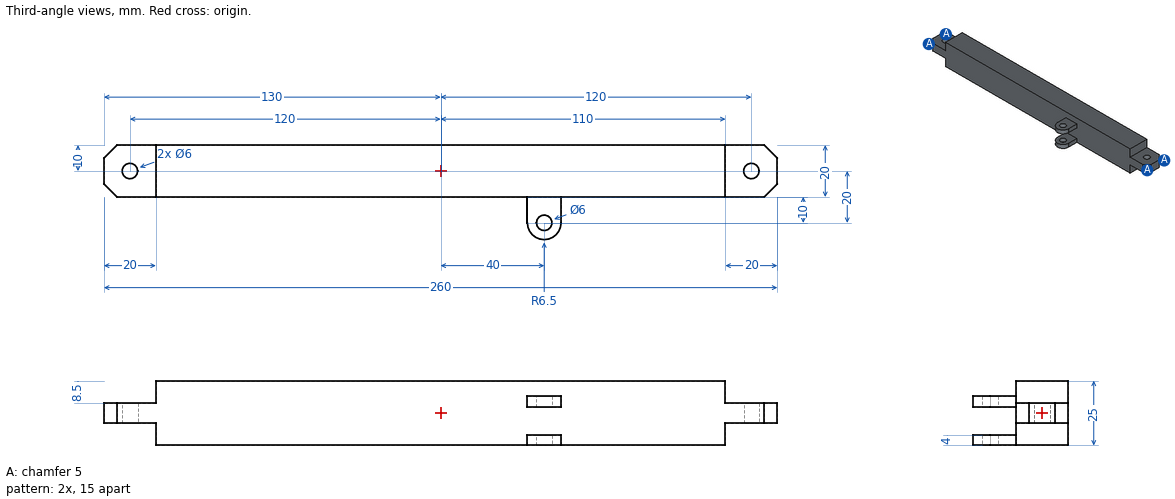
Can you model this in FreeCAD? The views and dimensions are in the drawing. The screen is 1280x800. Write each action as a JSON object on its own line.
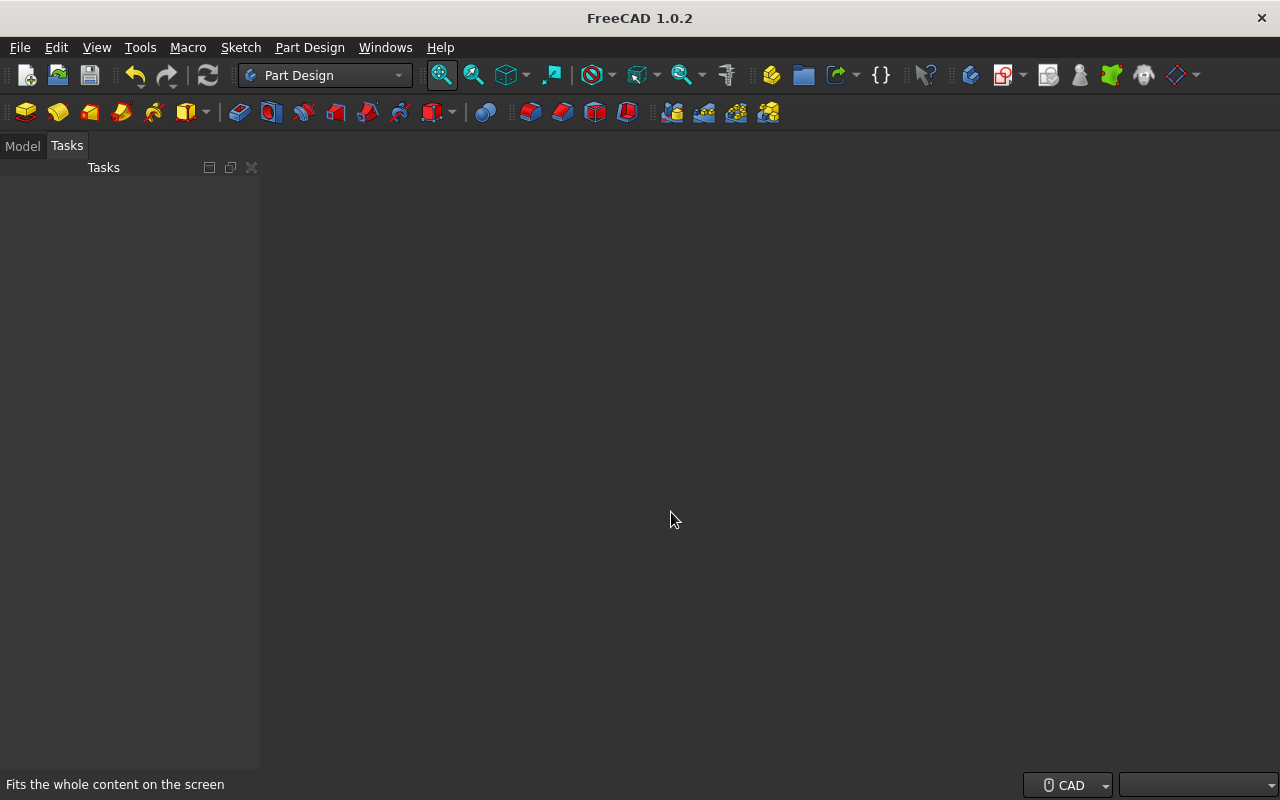
{"action": "key", "text": "ctrl+n"}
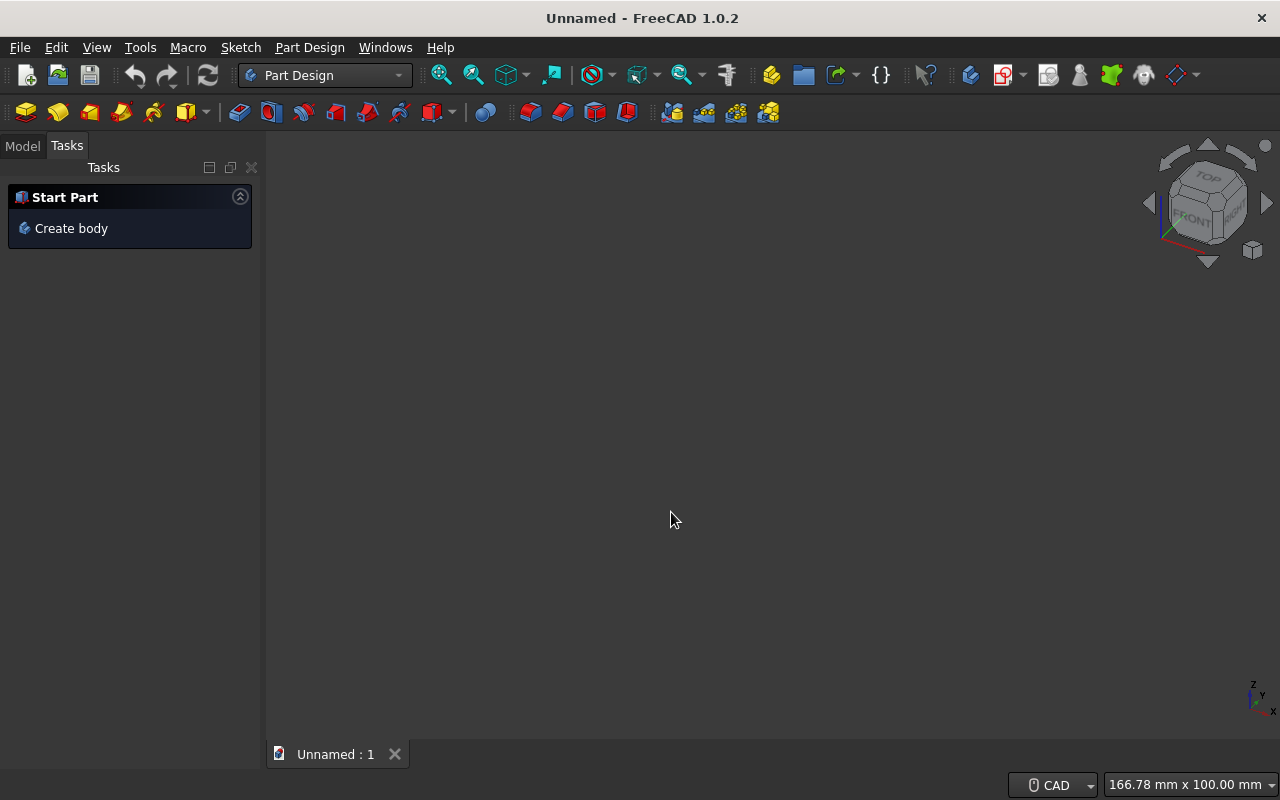
{"action": "left_click", "coordinate": [1004, 76]}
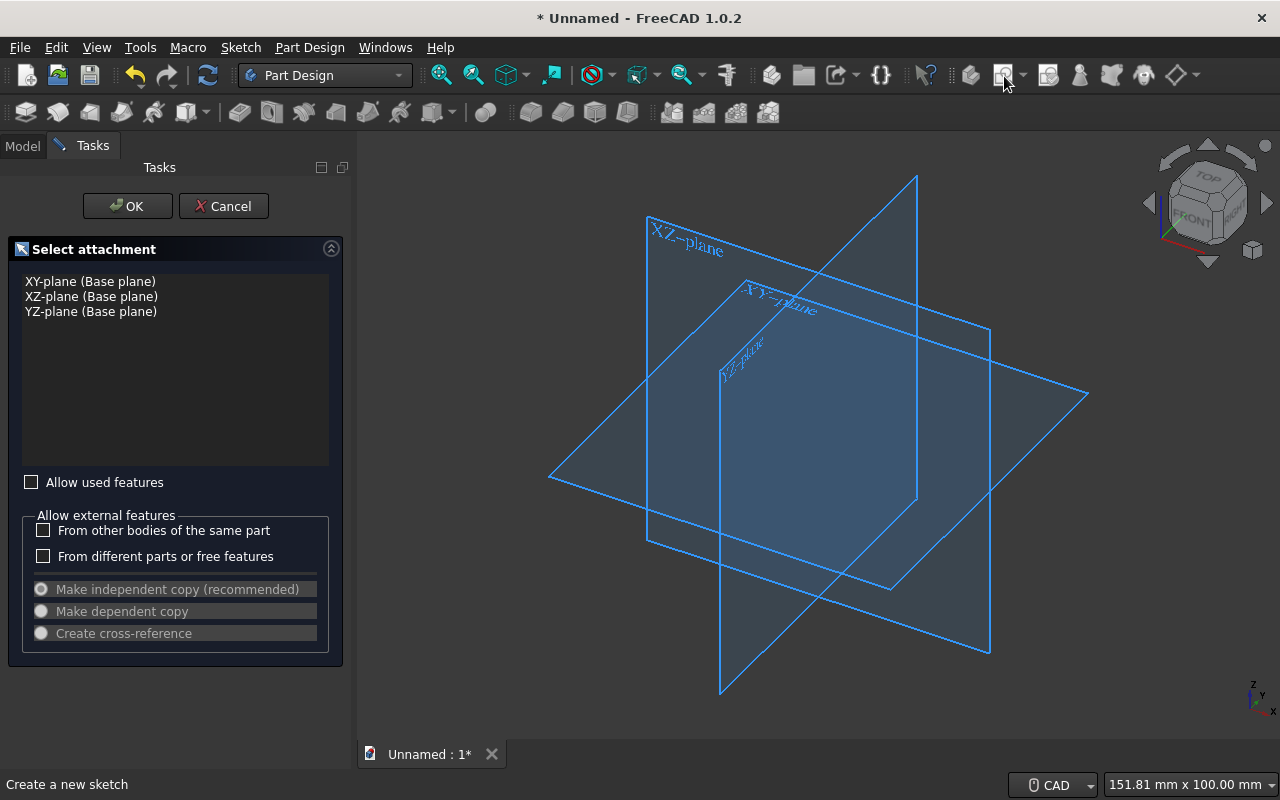
{"action": "left_click", "coordinate": [82, 282]}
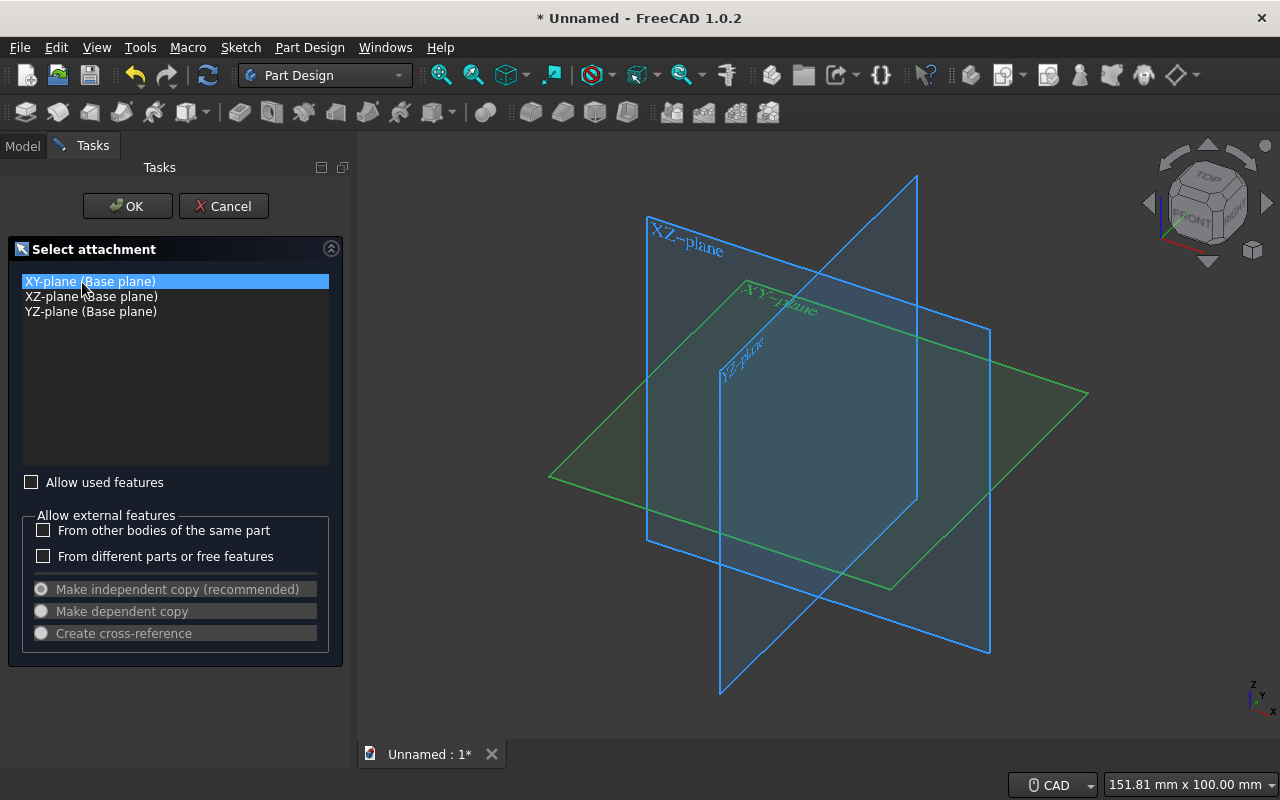
{"action": "left_click", "coordinate": [128, 206]}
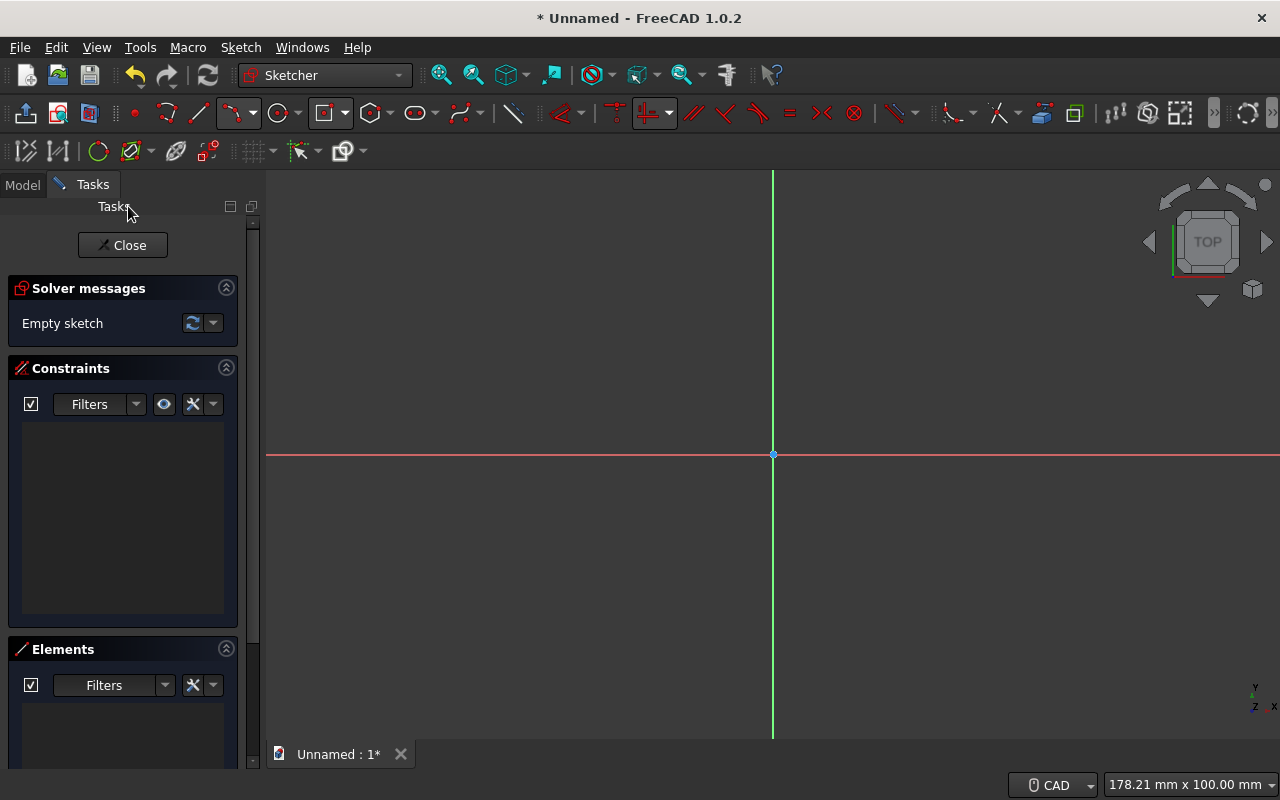
{"action": "scroll", "coordinate": [665, 454], "scroll_direction": "down", "scroll_amount": 5}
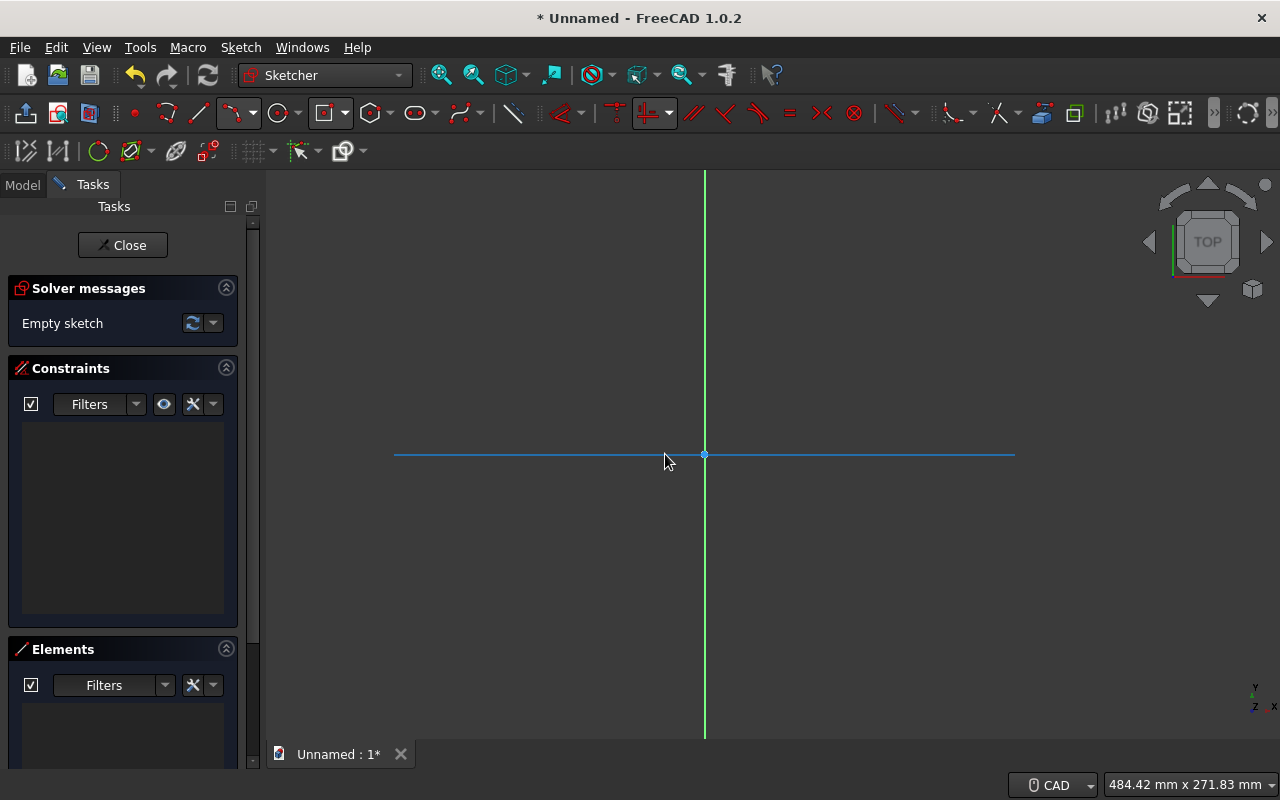
{"action": "key", "text": "g v"}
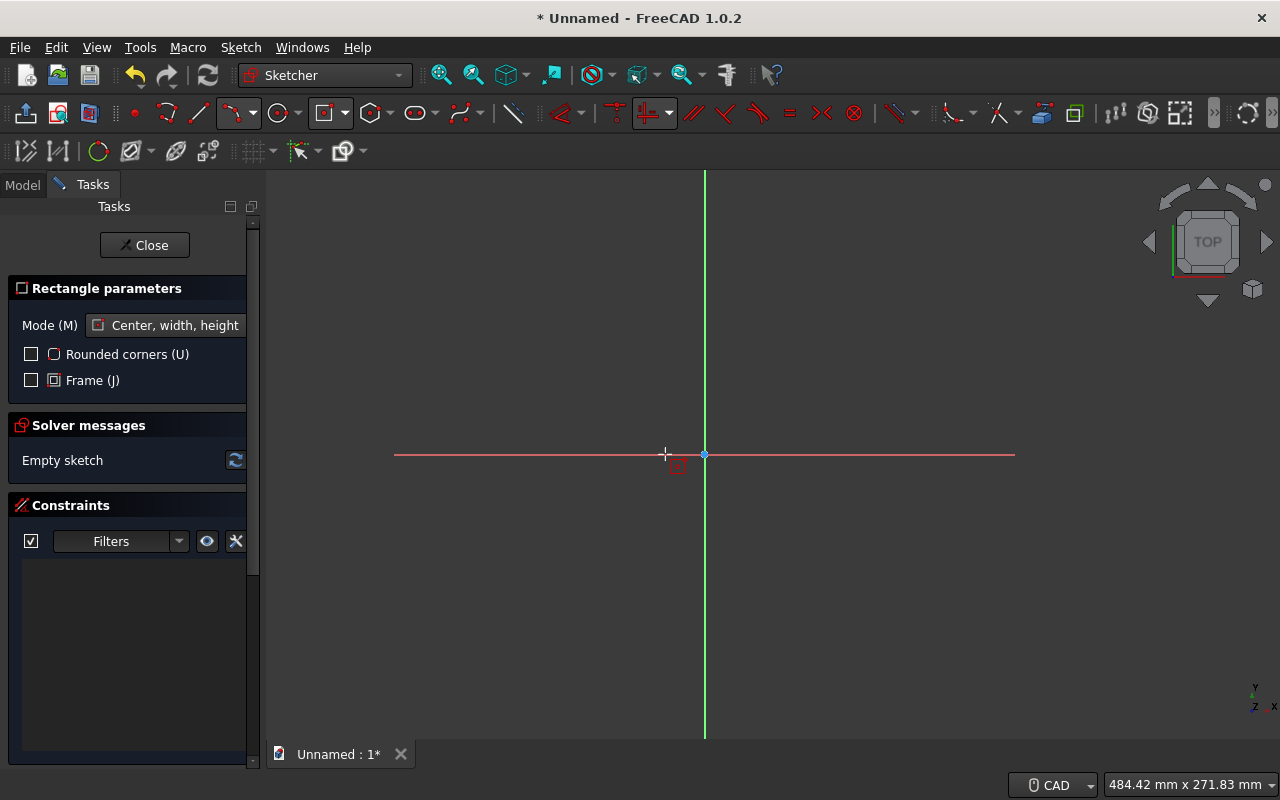
{"action": "left_click", "coordinate": [705, 454]}
{"action": "mouse_move", "coordinate": [977, 434]}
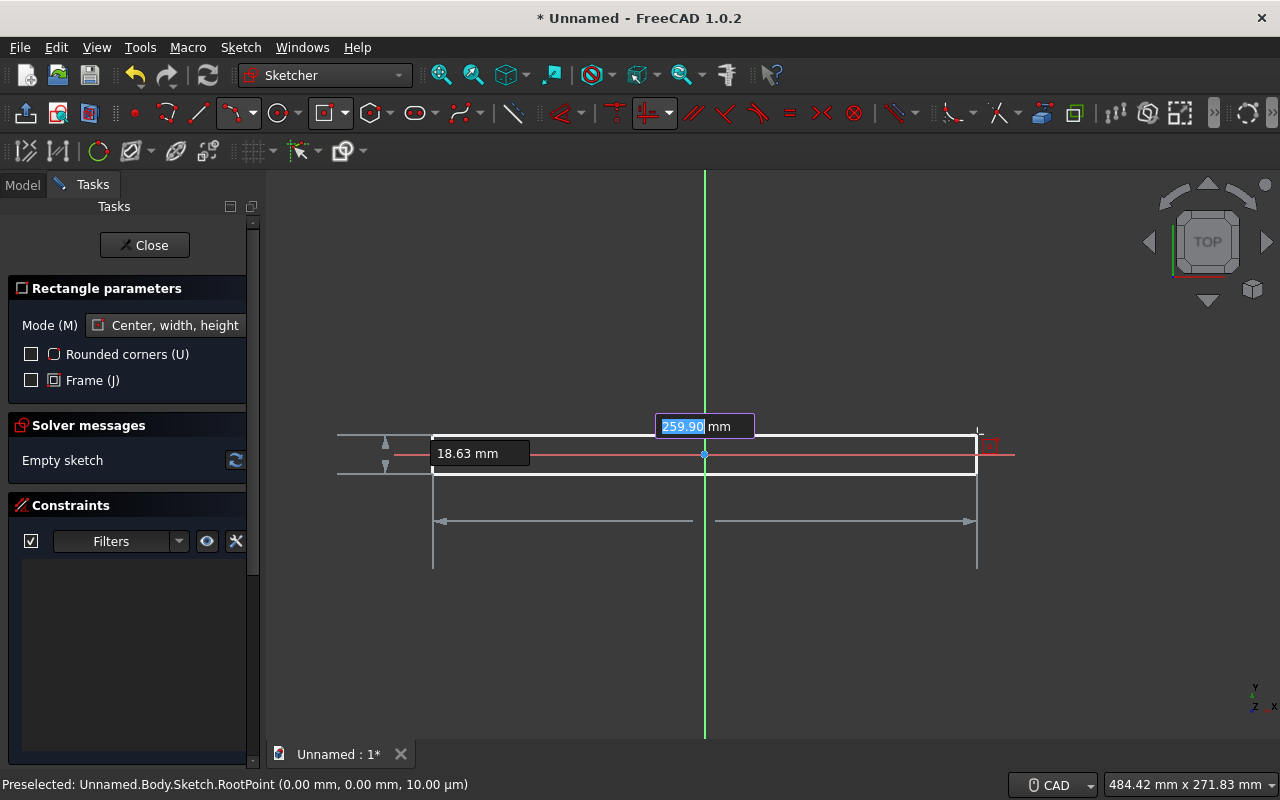
{"action": "type", "text": "260"}
{"action": "key", "text": "Tab"}
{"action": "type", "text": "20"}
{"action": "key", "text": "Return"}
{"action": "key", "text": "Escape"}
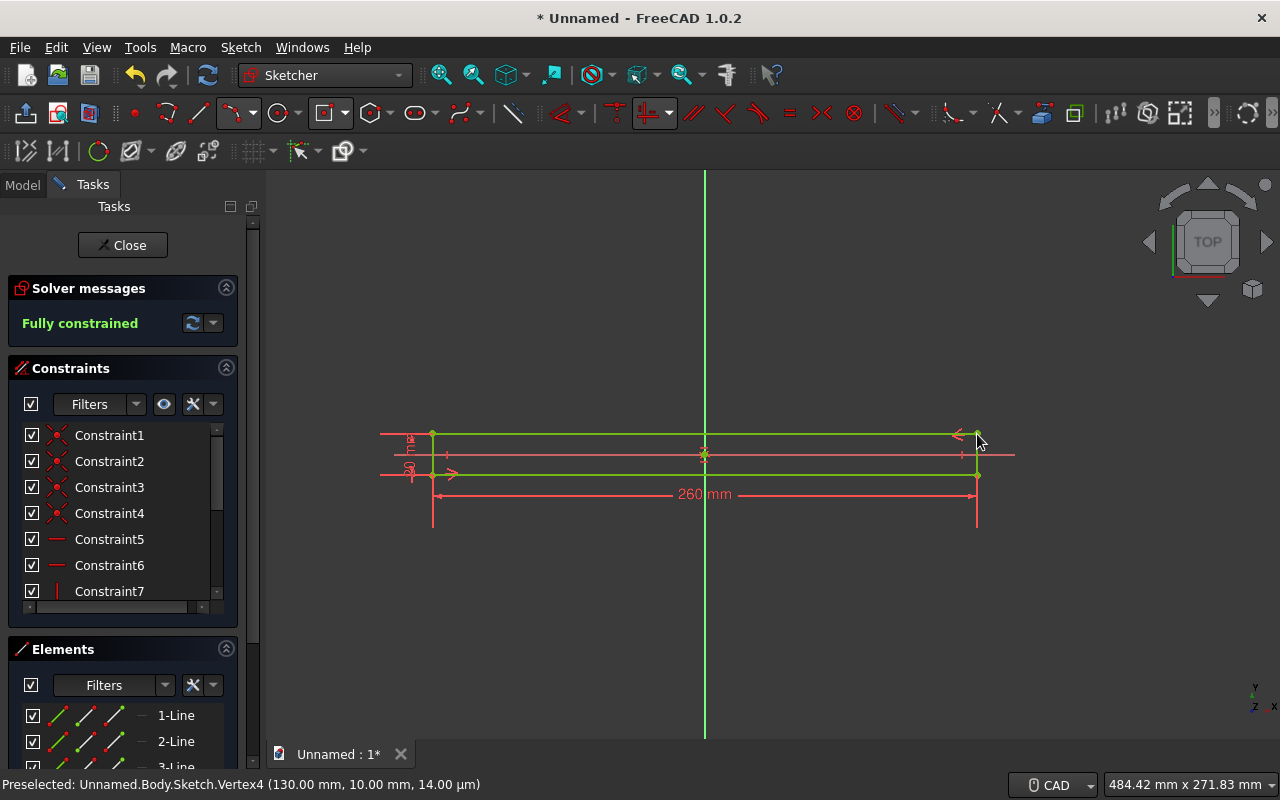
{"action": "left_click", "coordinate": [123, 245]}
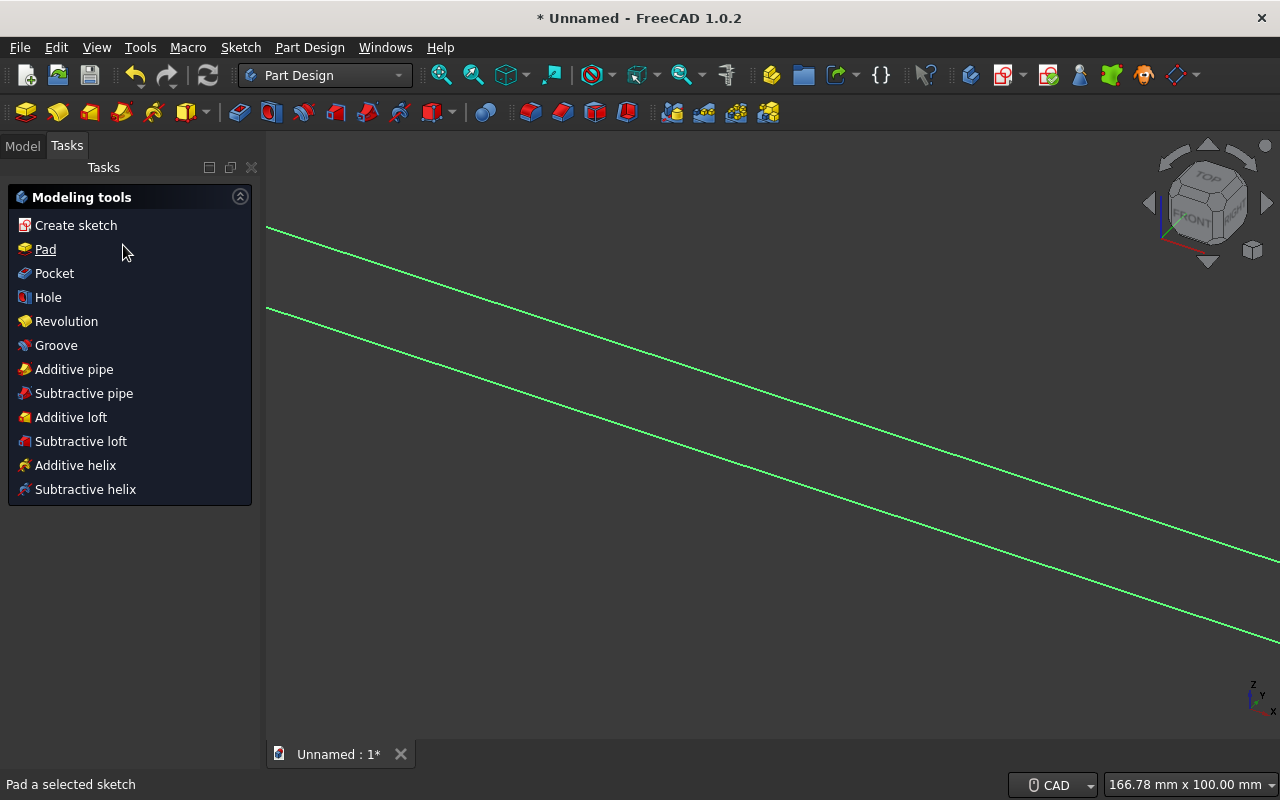
{"action": "left_click", "coordinate": [26, 112]}